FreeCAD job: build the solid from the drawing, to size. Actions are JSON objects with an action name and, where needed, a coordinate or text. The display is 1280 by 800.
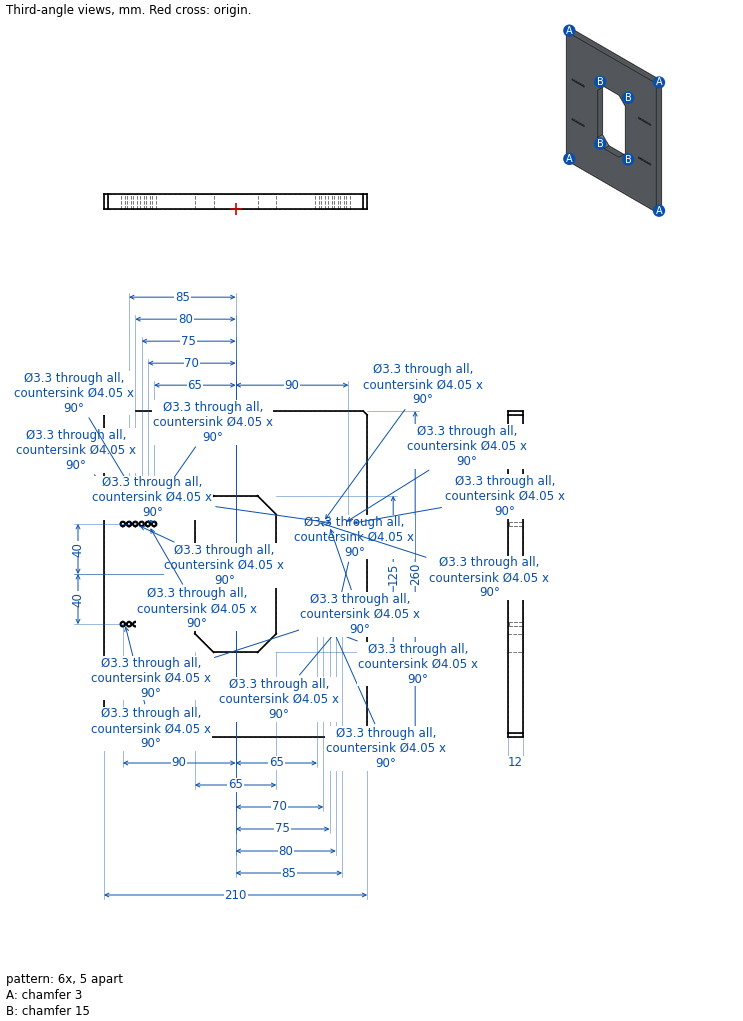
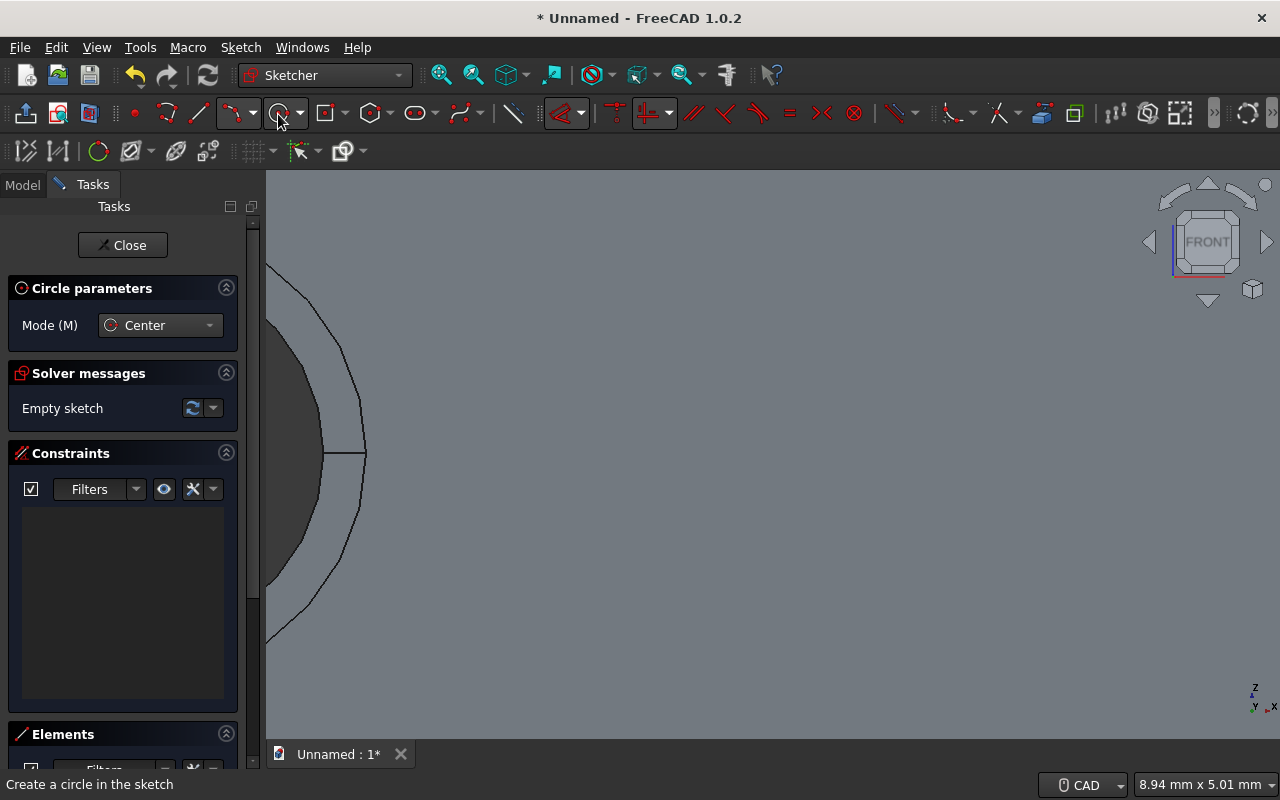
{"action": "left_click", "coordinate": [704, 453]}
{"action": "mouse_move", "coordinate": [836, 321]}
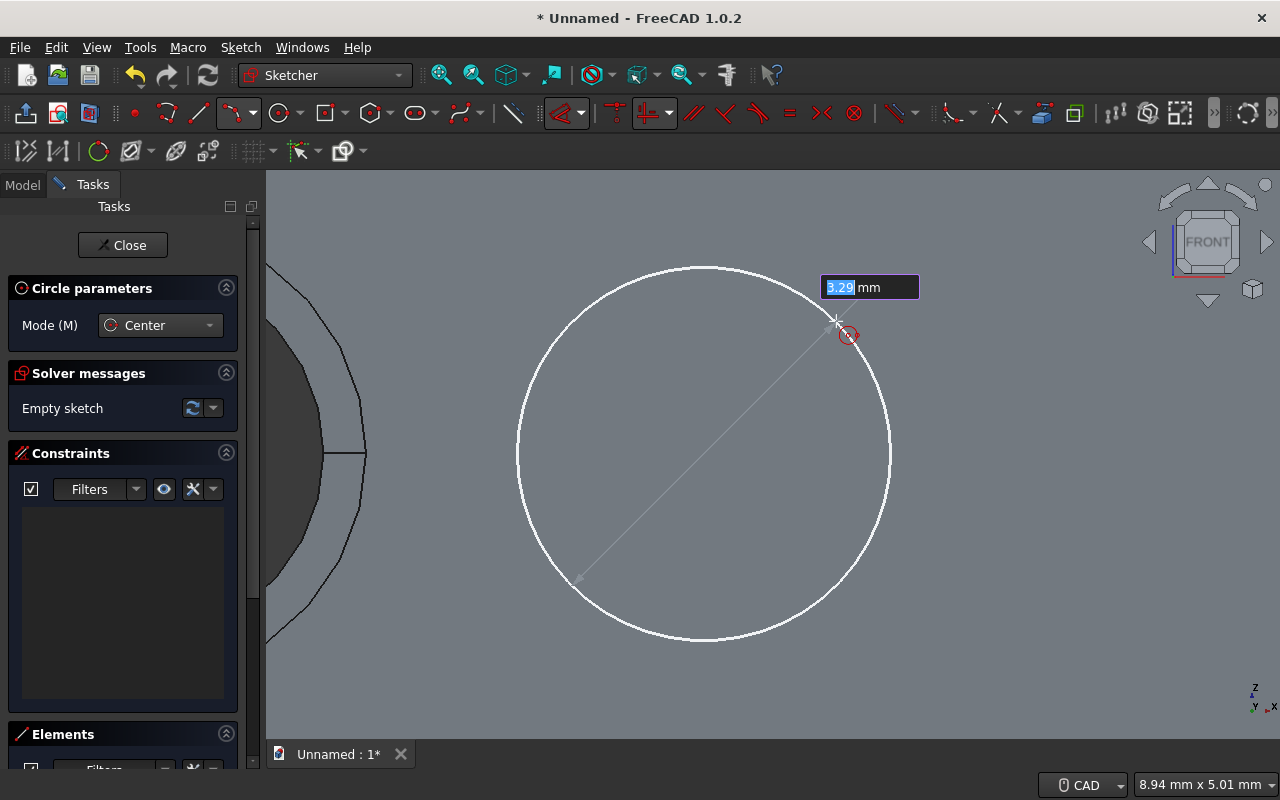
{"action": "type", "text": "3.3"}
{"action": "key", "text": "Return"}
{"action": "key", "text": "Escape"}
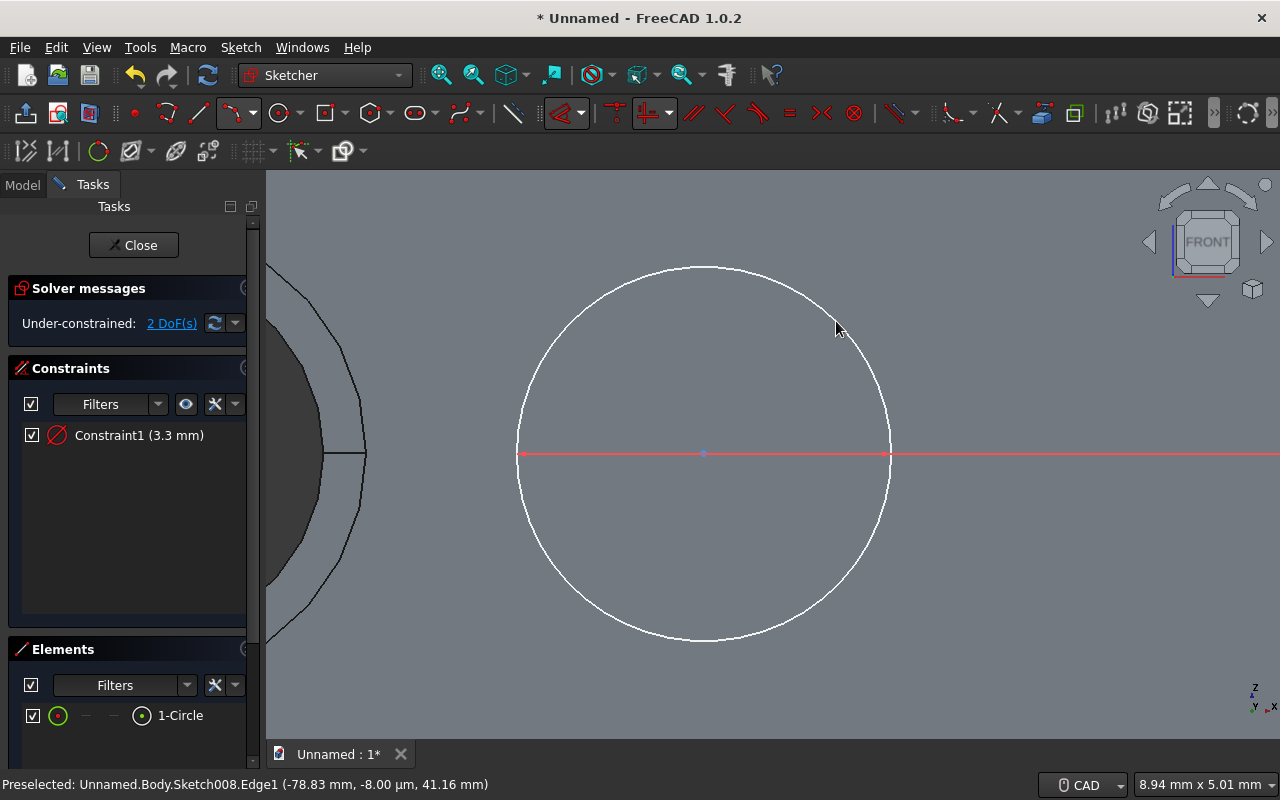
{"action": "left_click", "coordinate": [704, 454]}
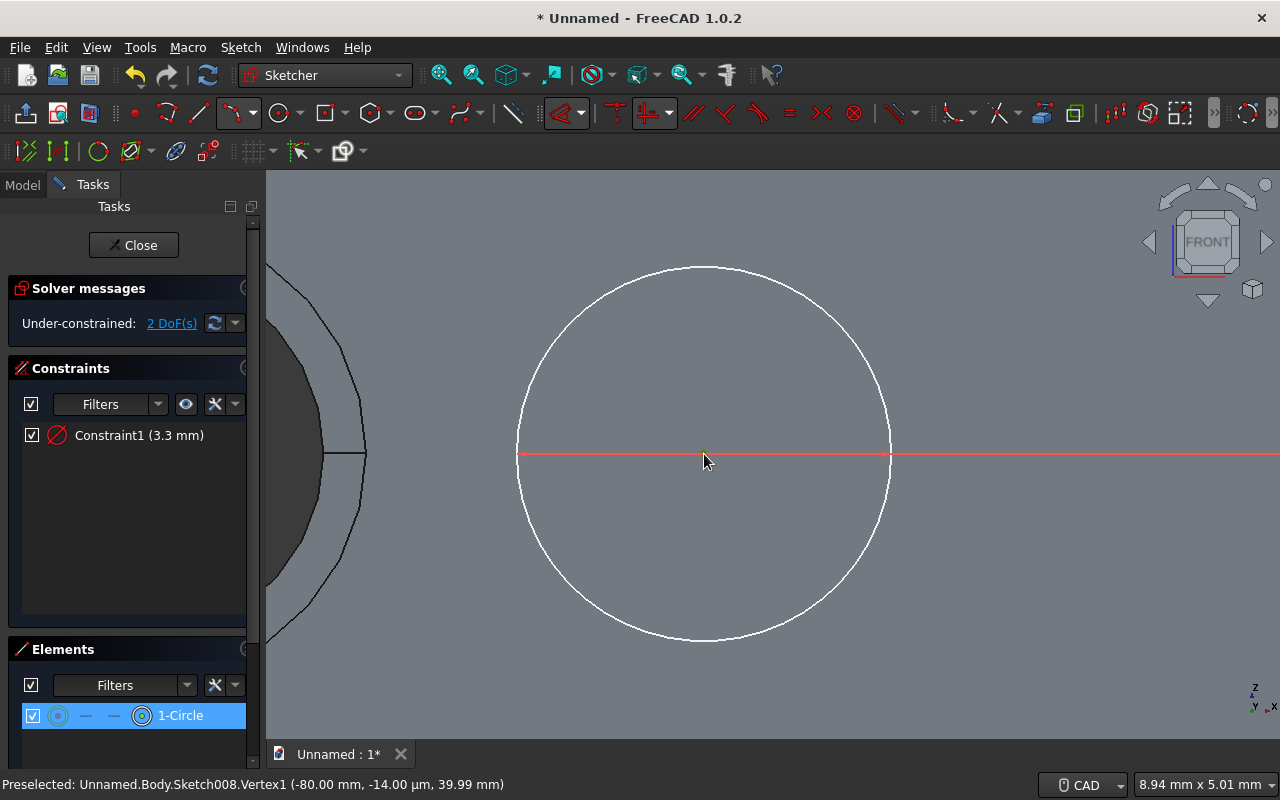
{"action": "key", "text": "l"}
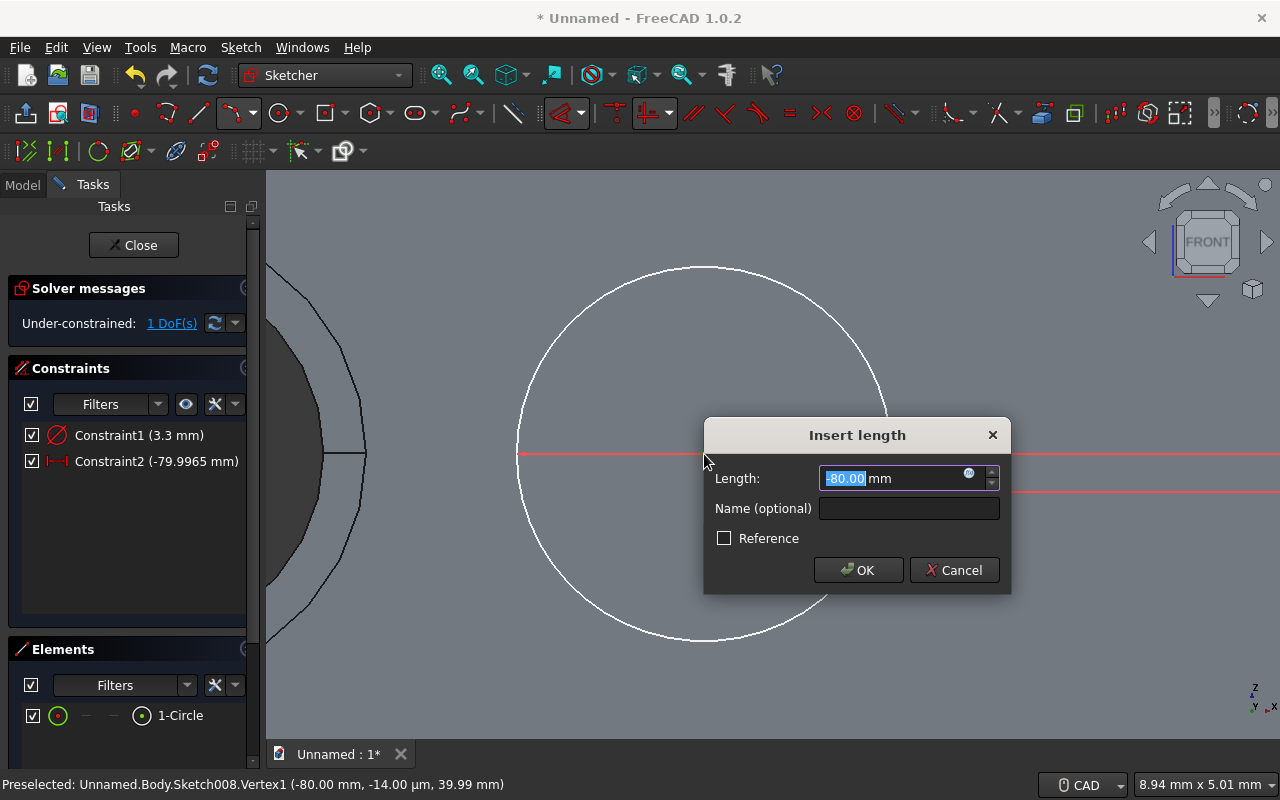
{"action": "type", "text": "-80"}
{"action": "key", "text": "Return"}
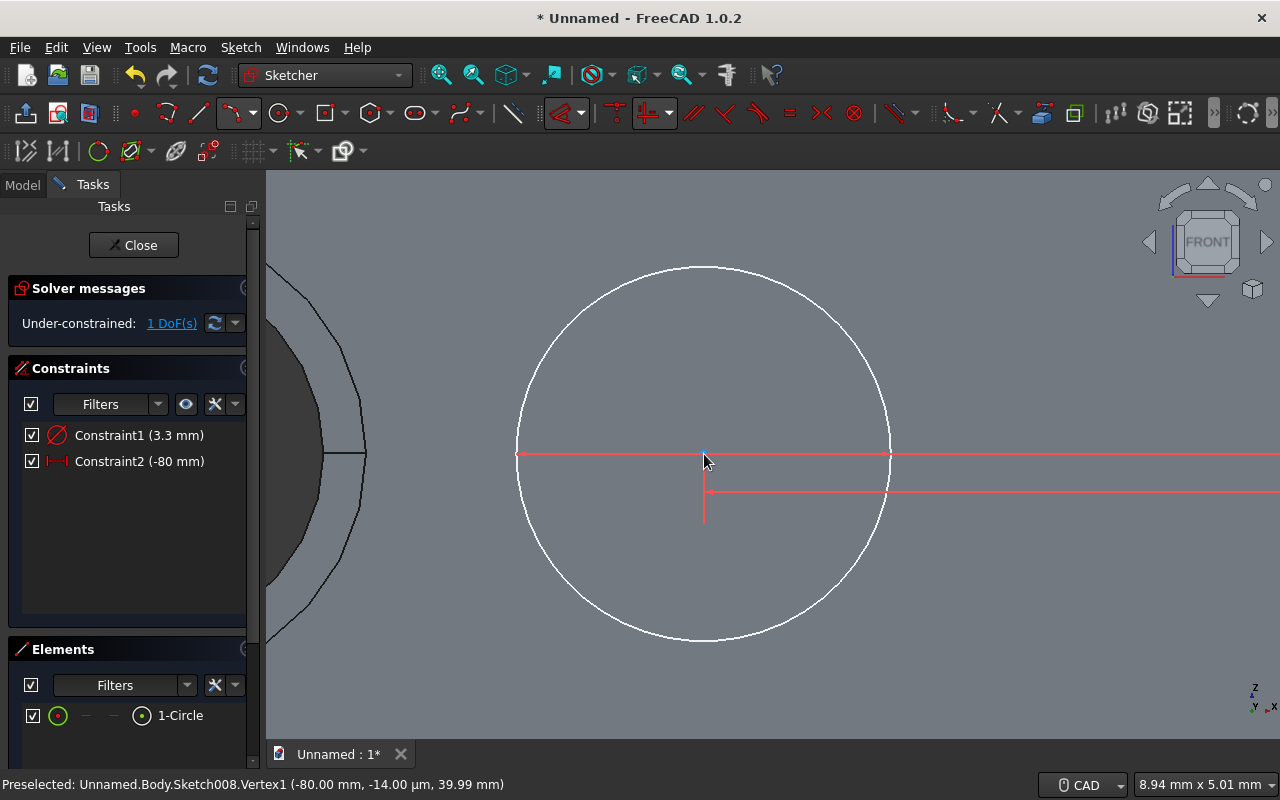
{"action": "left_click", "coordinate": [704, 454]}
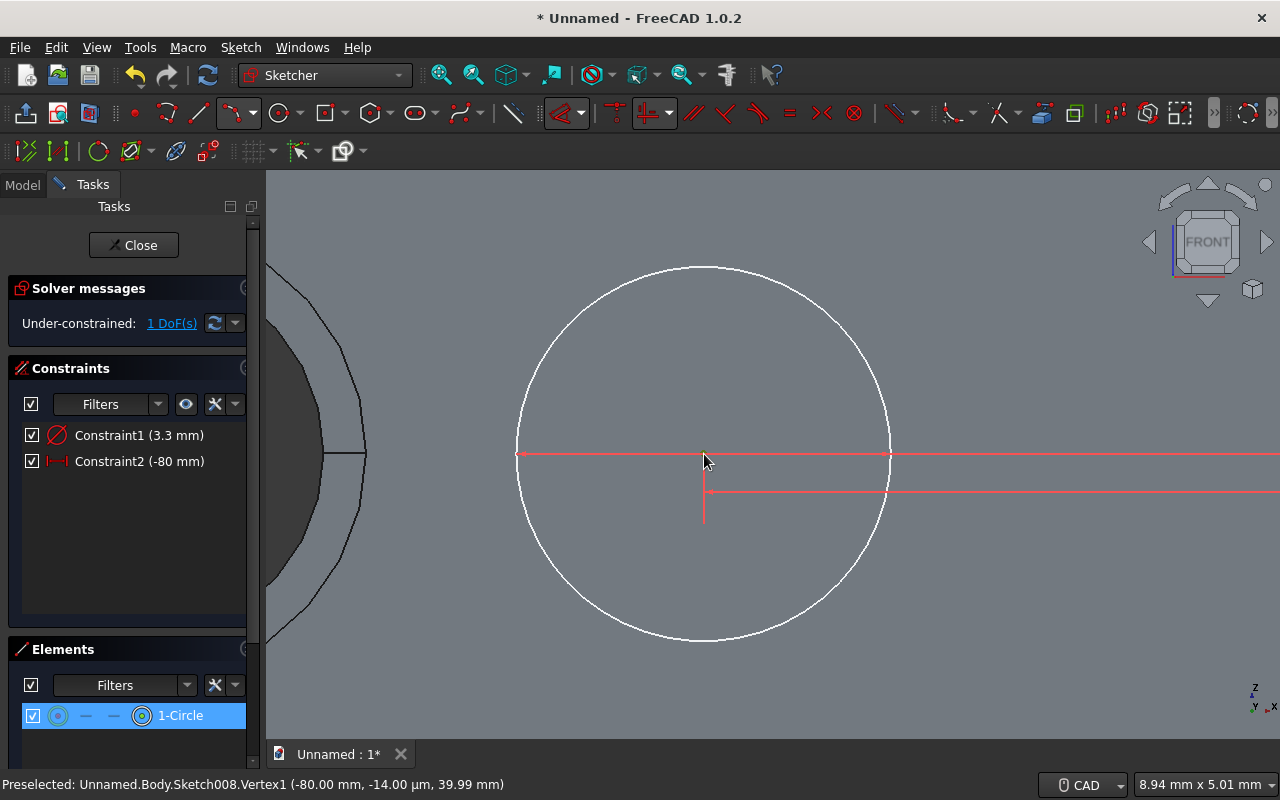
{"action": "left_click", "coordinate": [584, 114]}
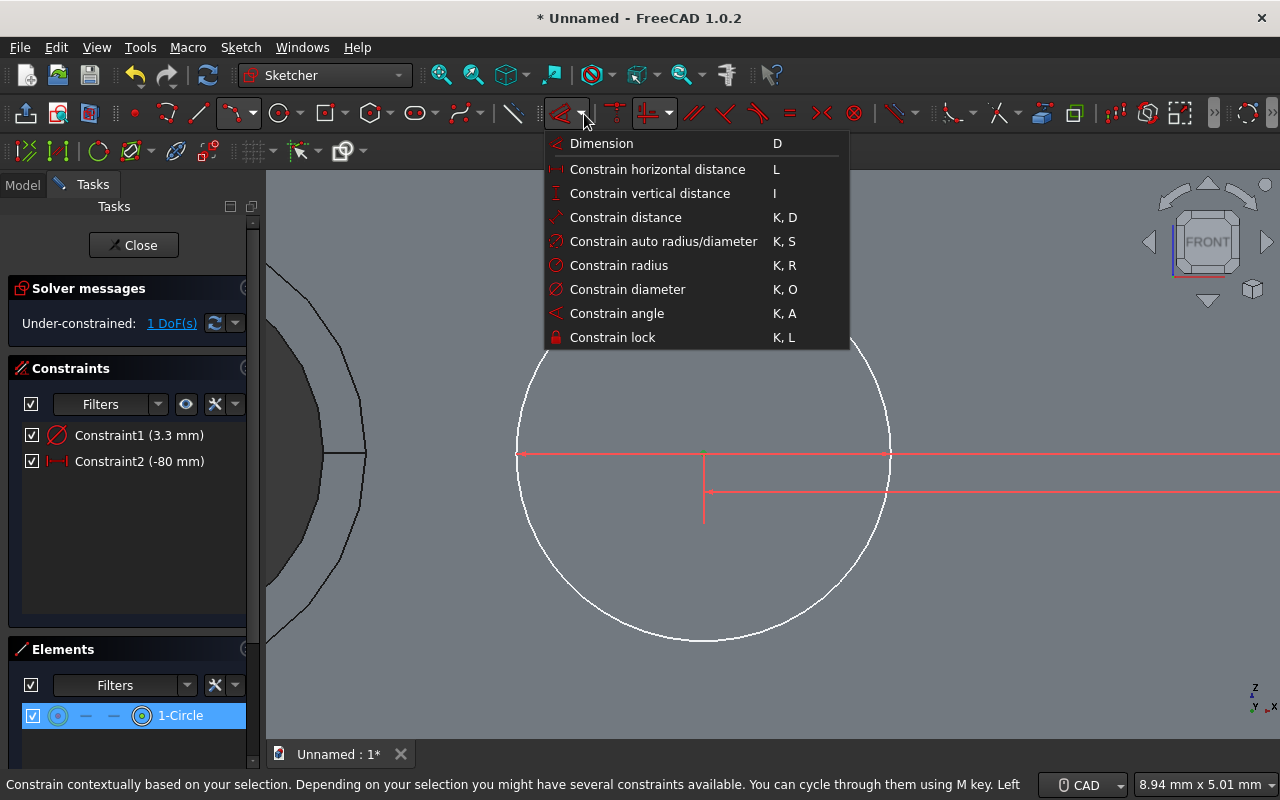
{"action": "left_click", "coordinate": [697, 193]}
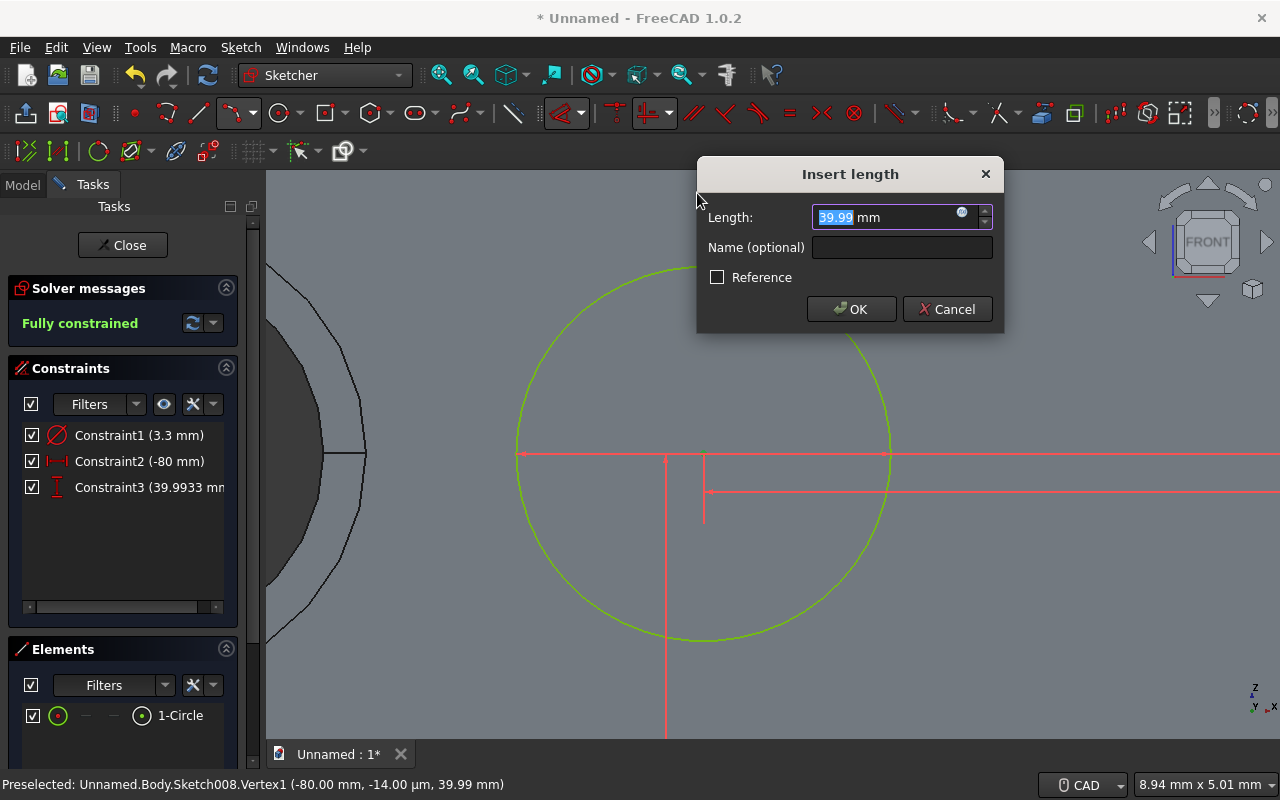
{"action": "type", "text": "40"}
{"action": "key", "text": "Return"}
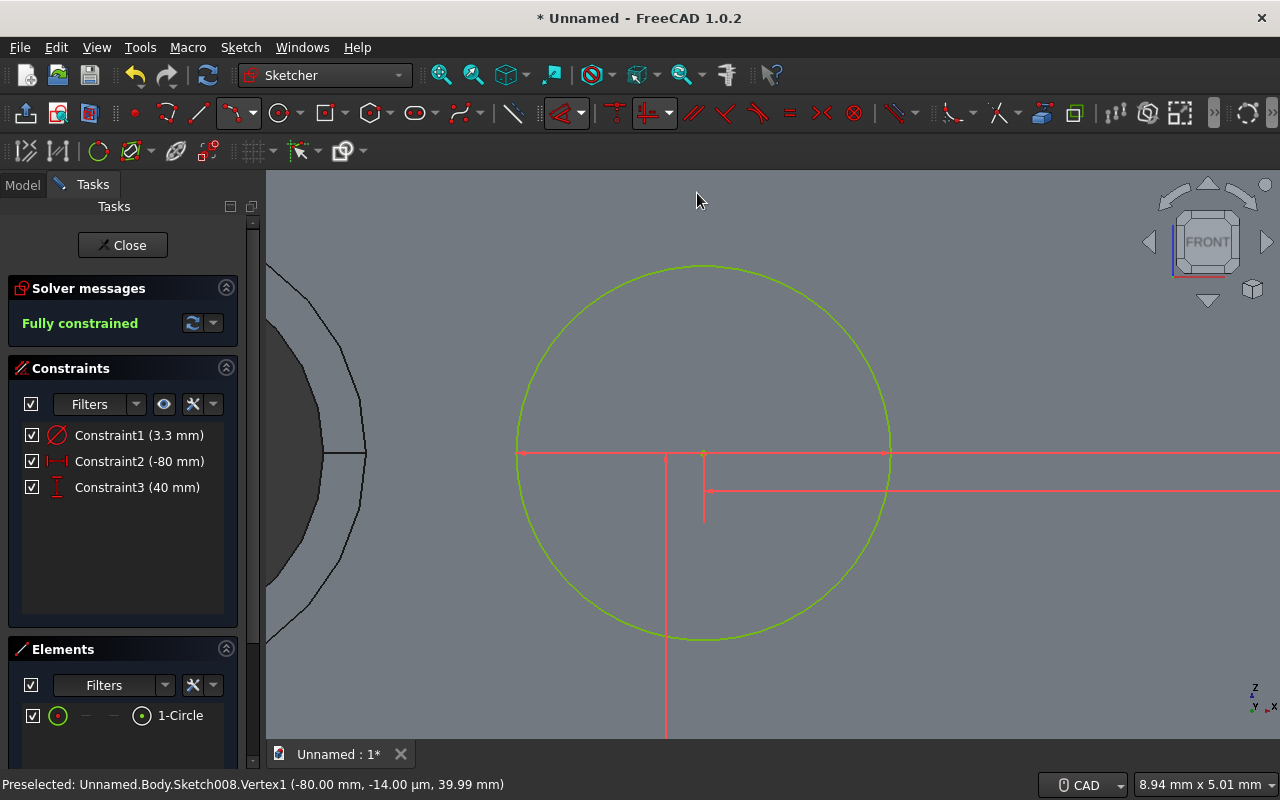
{"action": "left_click", "coordinate": [123, 245]}